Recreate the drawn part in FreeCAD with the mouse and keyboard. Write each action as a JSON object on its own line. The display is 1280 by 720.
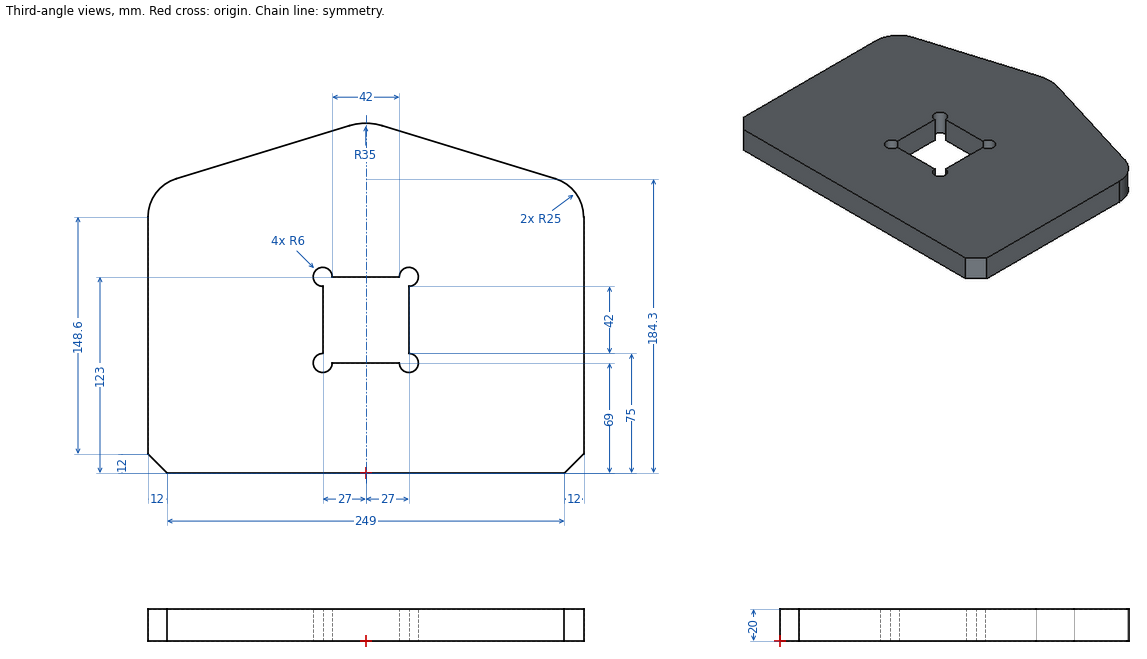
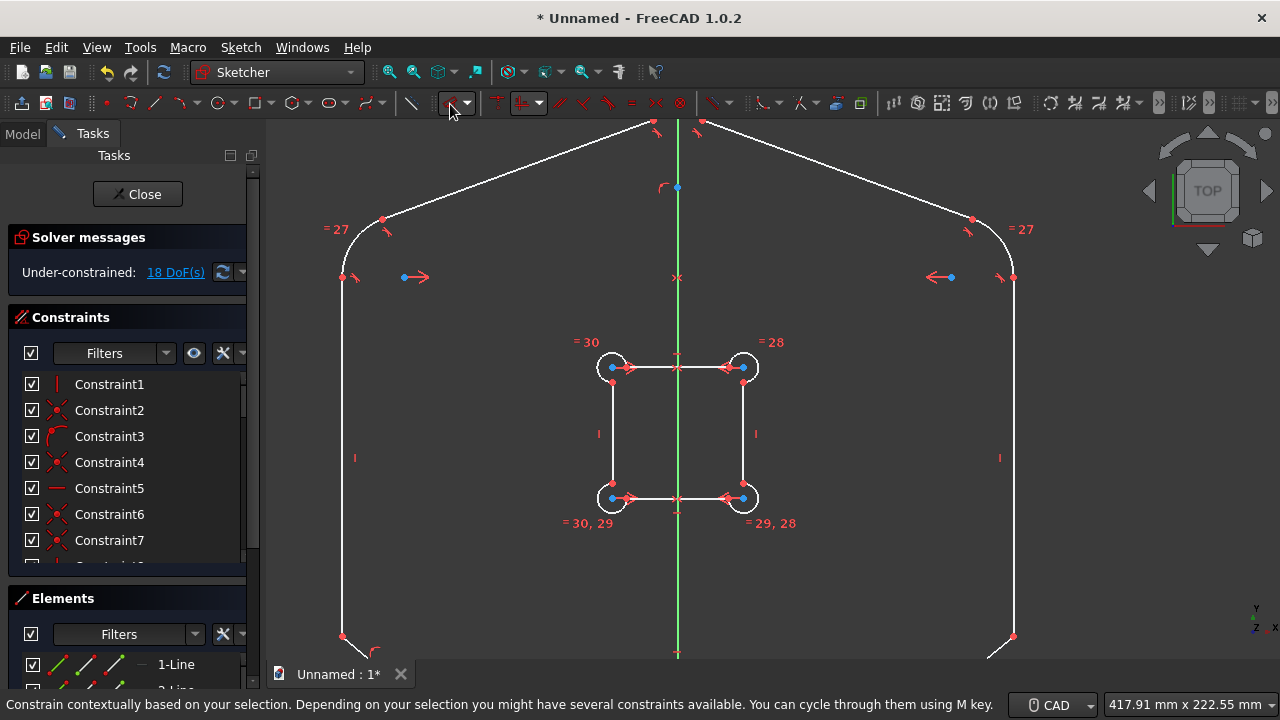
{"action": "scroll", "coordinate": [759, 369], "scroll_direction": "down", "scroll_amount": 2}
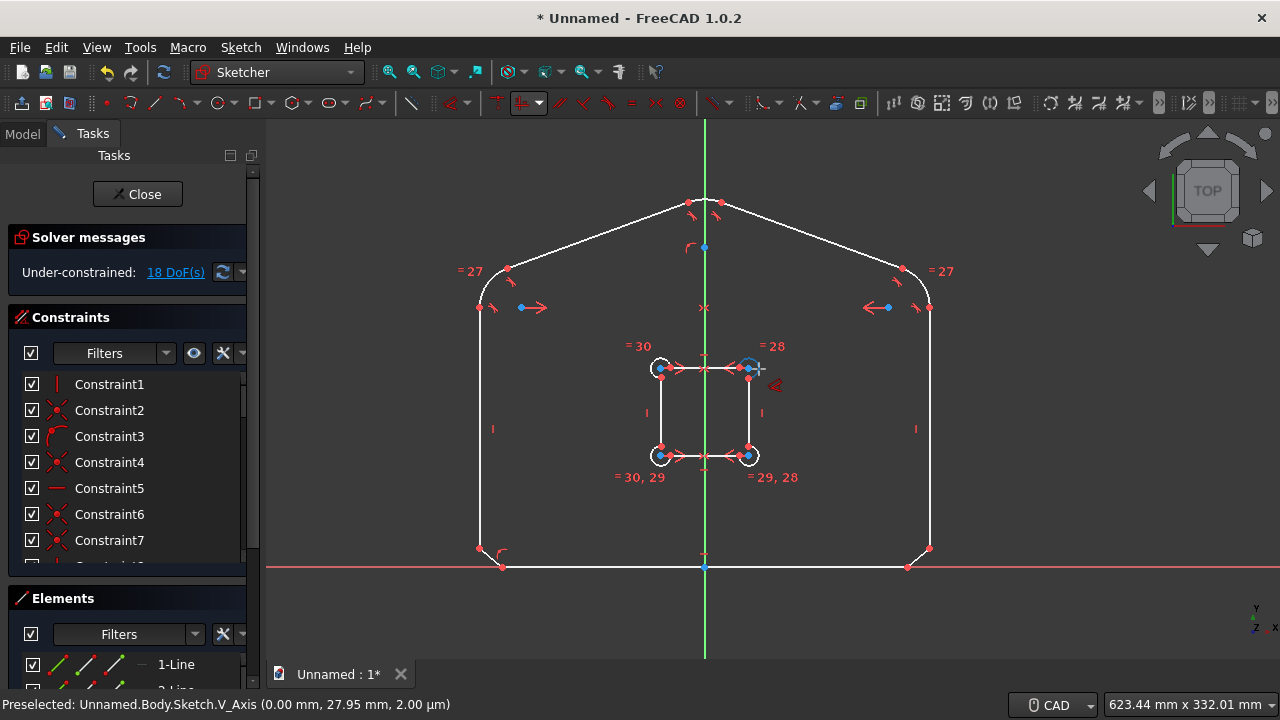
{"action": "scroll", "coordinate": [712, 200], "scroll_direction": "up", "scroll_amount": 4}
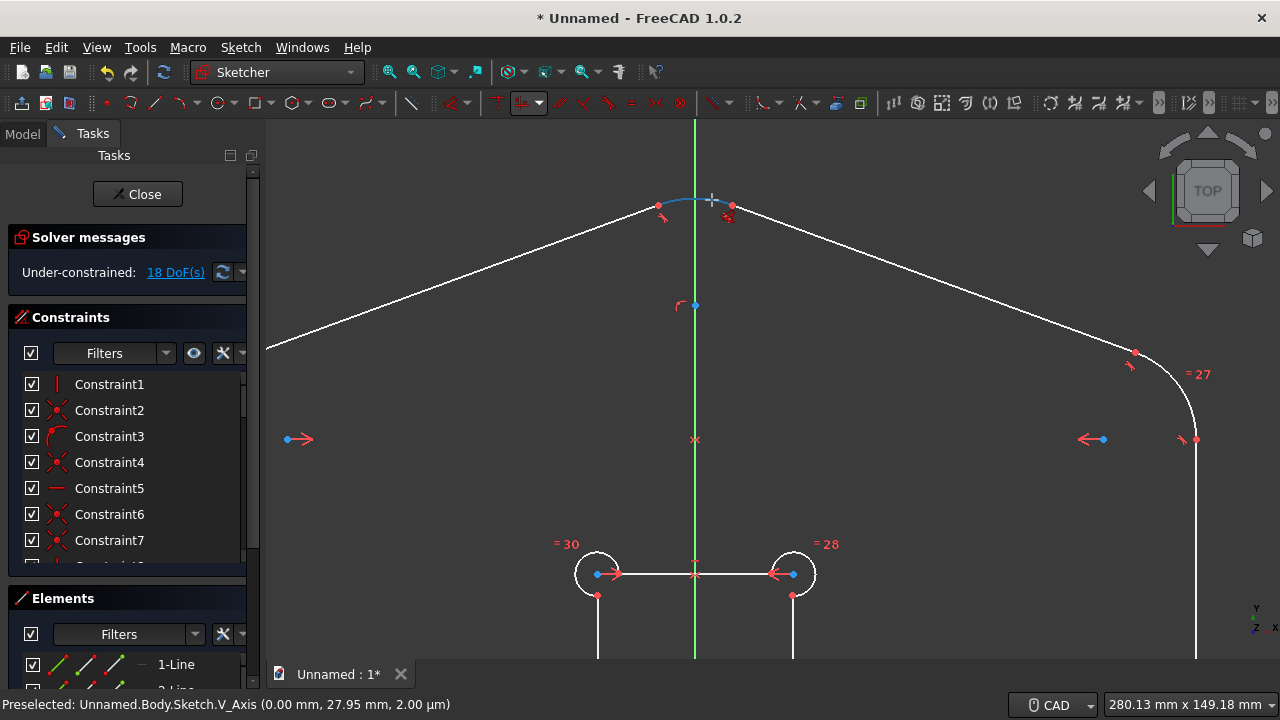
{"action": "left_click", "coordinate": [710, 200]}
{"action": "left_click", "coordinate": [714, 168]}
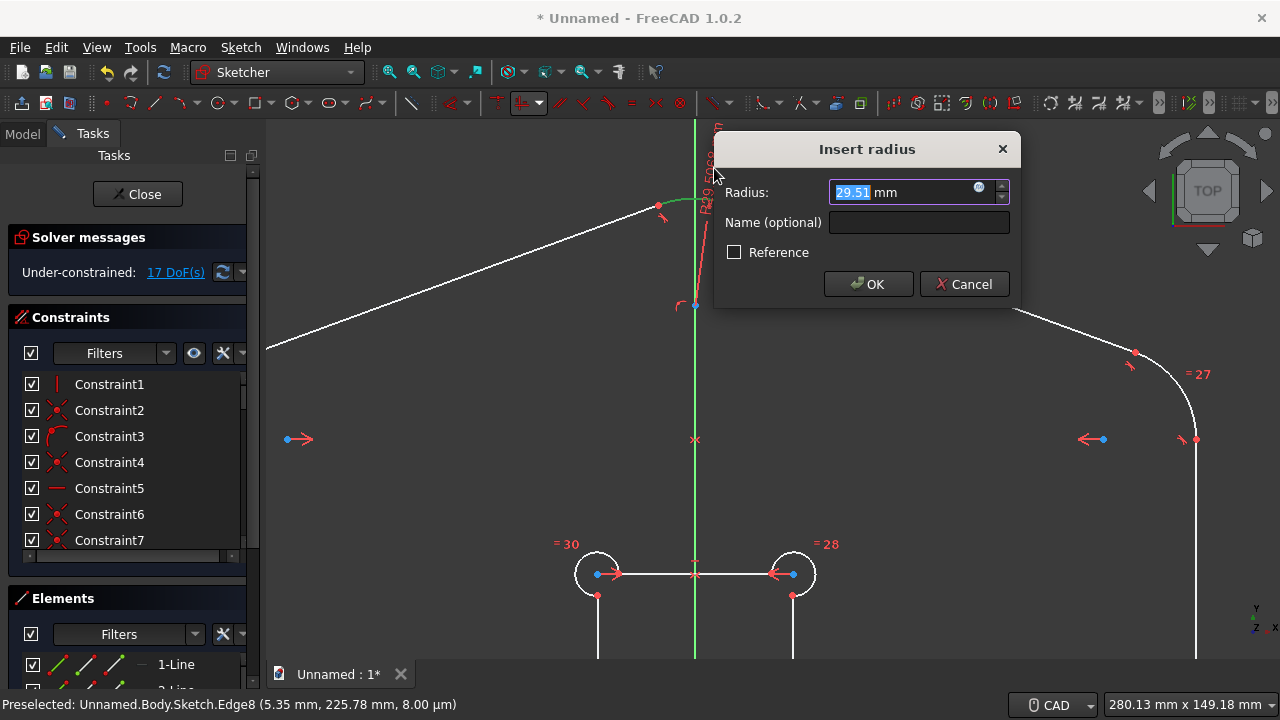
{"action": "type", "text": "35"}
{"action": "key", "text": "Return"}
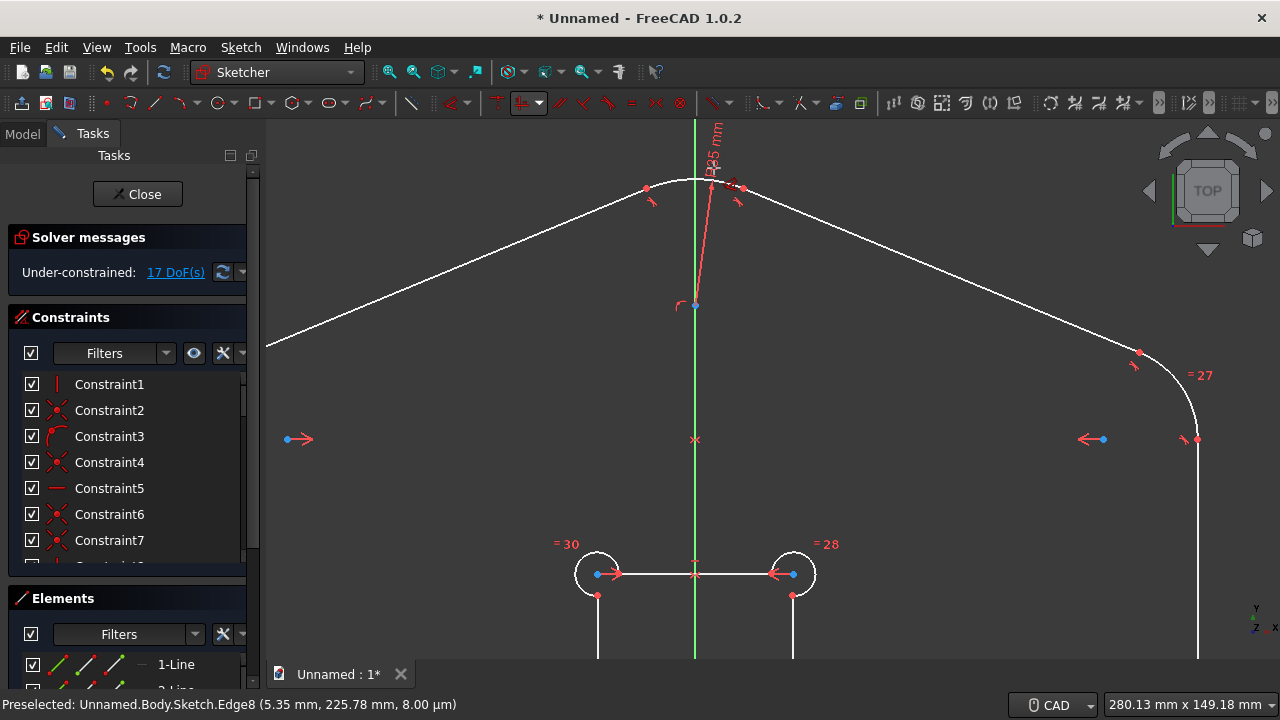
{"action": "scroll", "coordinate": [712, 200], "scroll_direction": "down", "scroll_amount": 4}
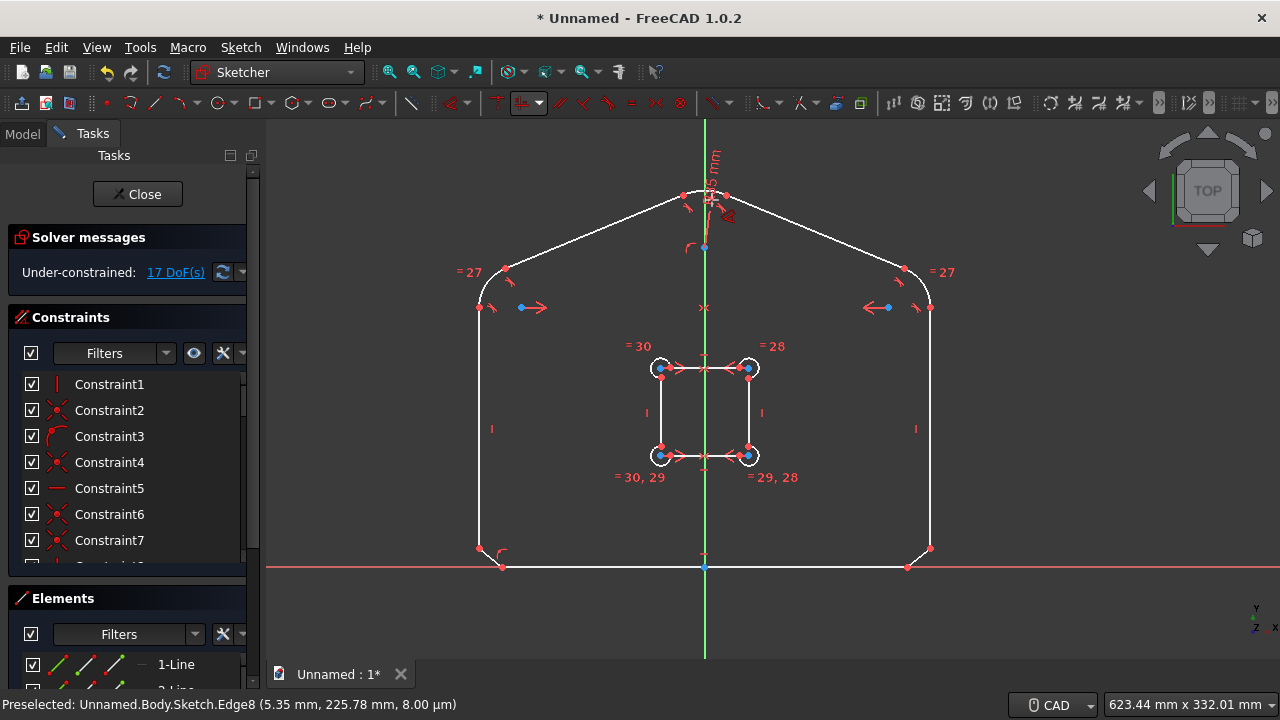
{"action": "left_click", "coordinate": [493, 277]}
{"action": "left_click", "coordinate": [471, 253]}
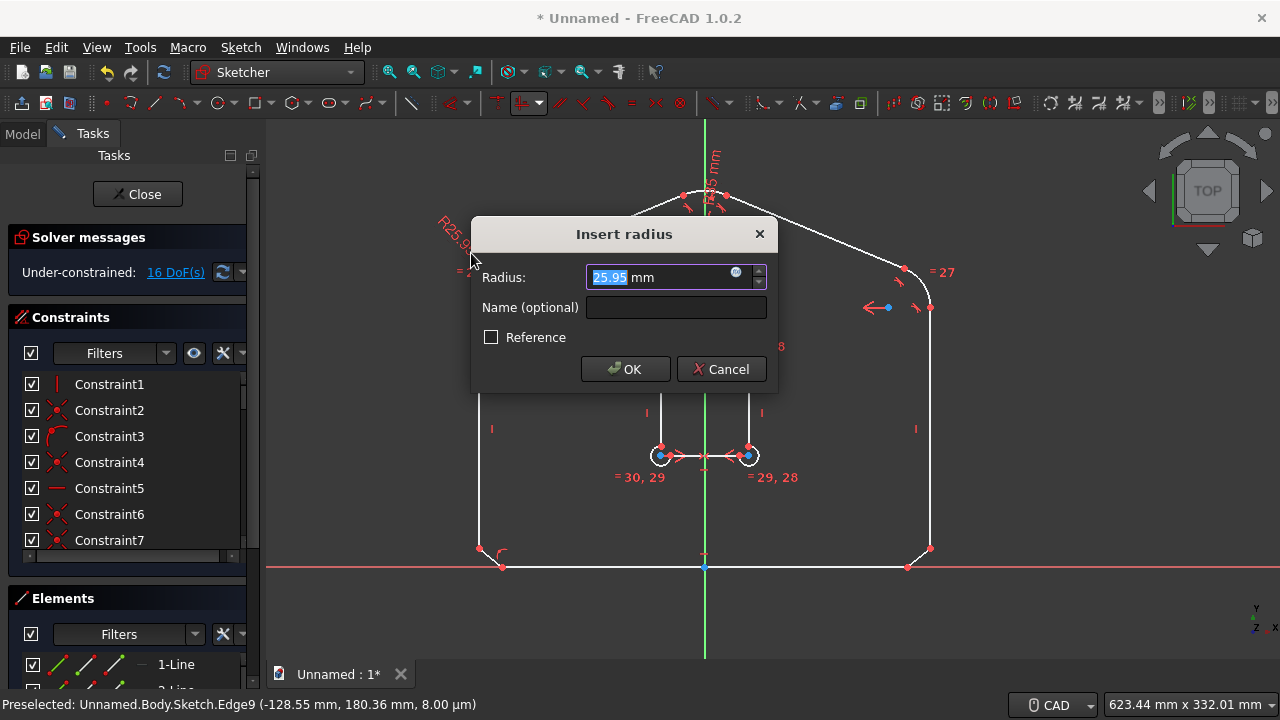
{"action": "type", "text": "25"}
{"action": "key", "text": "Return"}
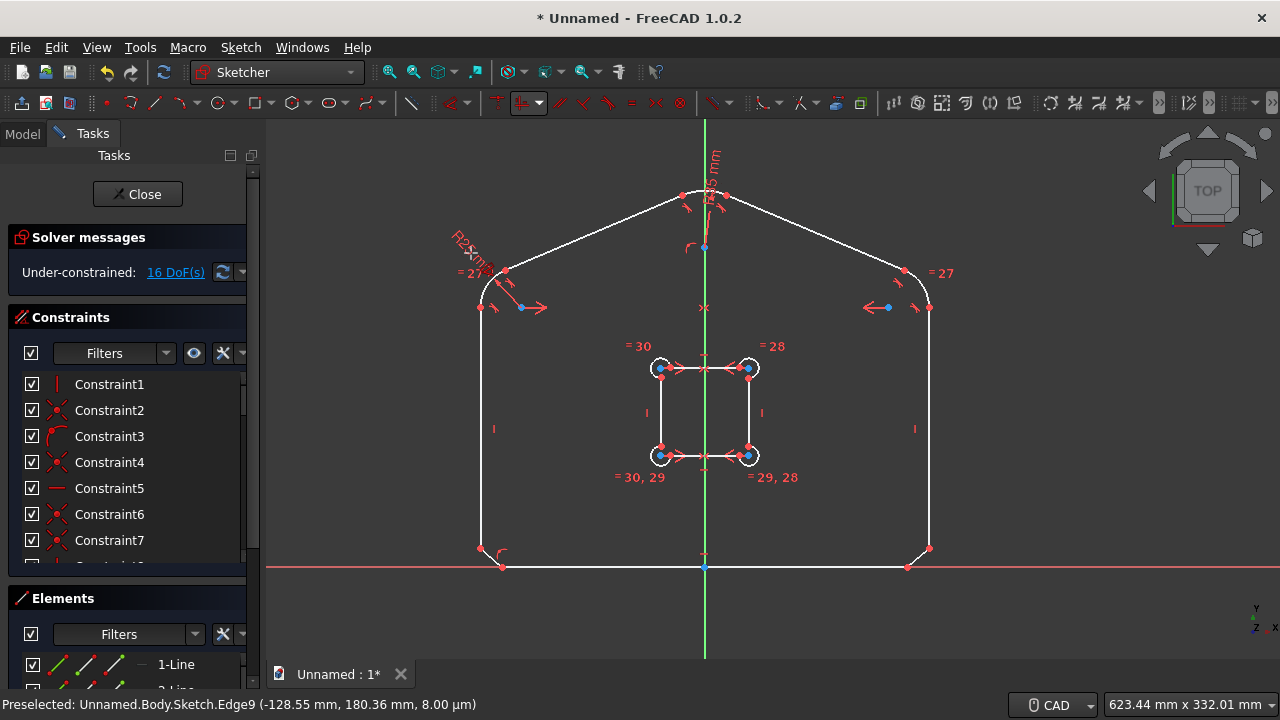
{"action": "scroll", "coordinate": [759, 370], "scroll_direction": "up", "scroll_amount": 8}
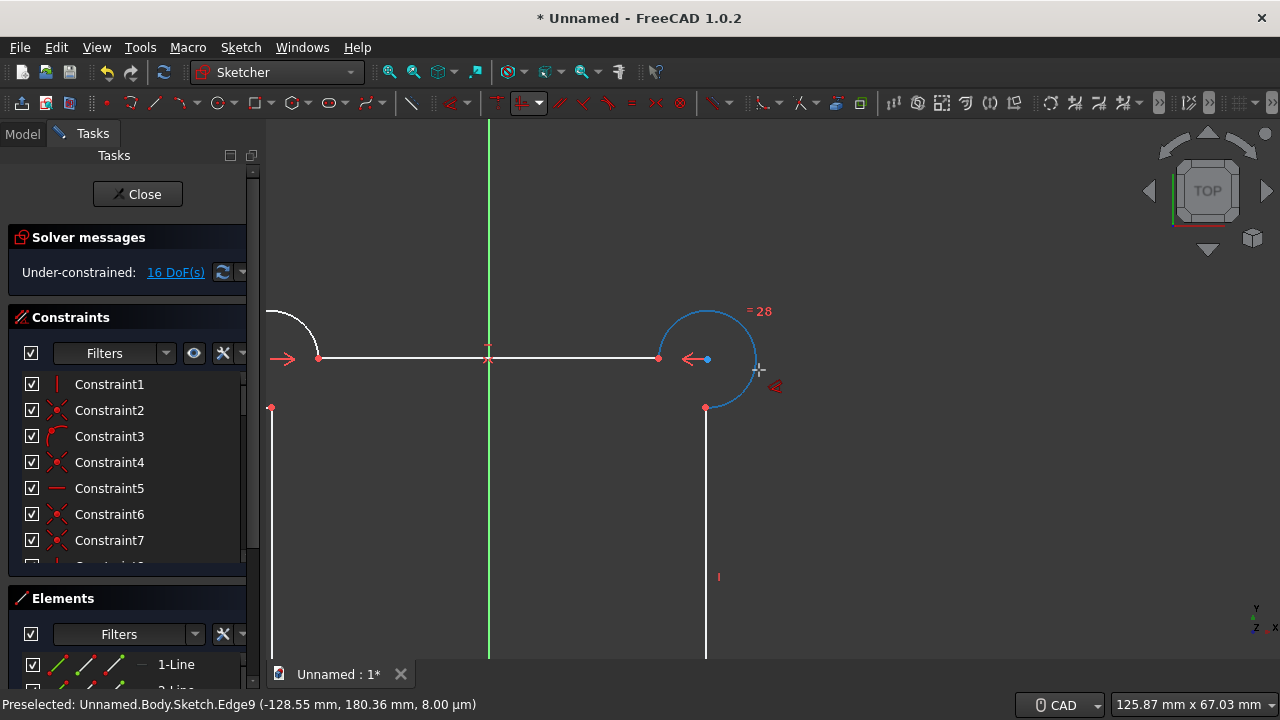
{"action": "left_click", "coordinate": [755, 368]}
{"action": "left_click", "coordinate": [786, 374]}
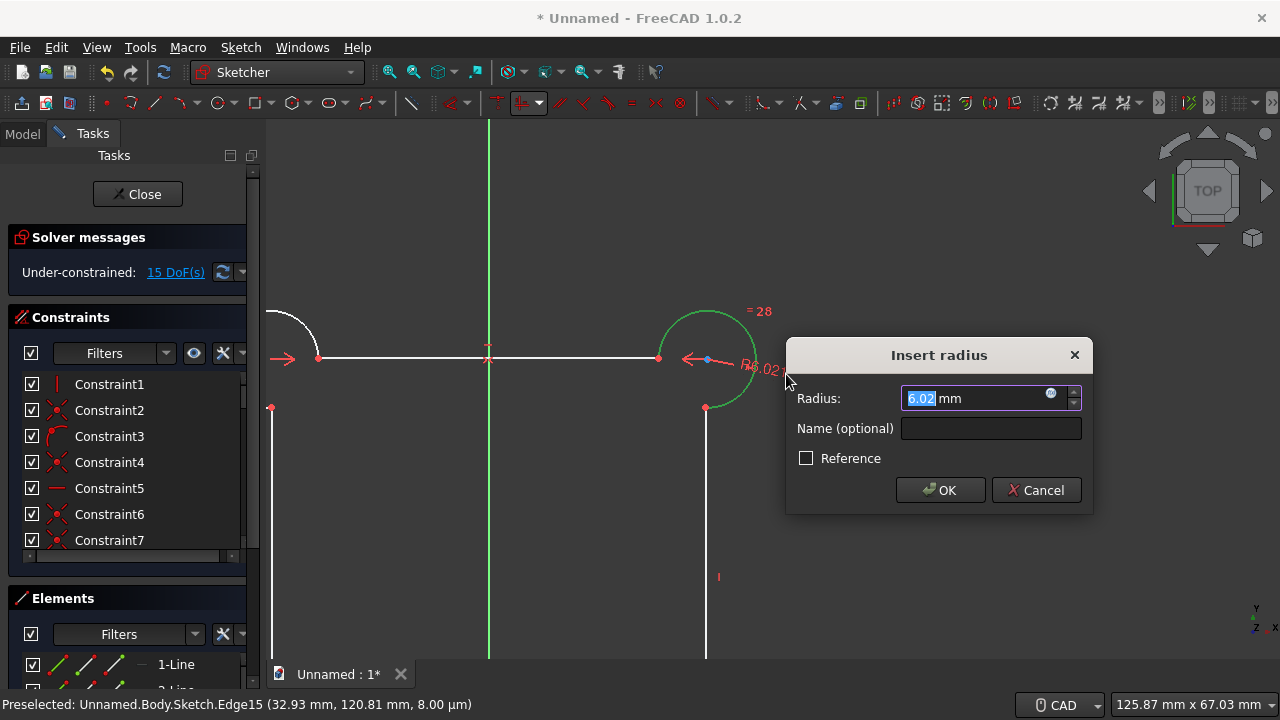
{"action": "type", "text": "6"}
{"action": "key", "text": "Return"}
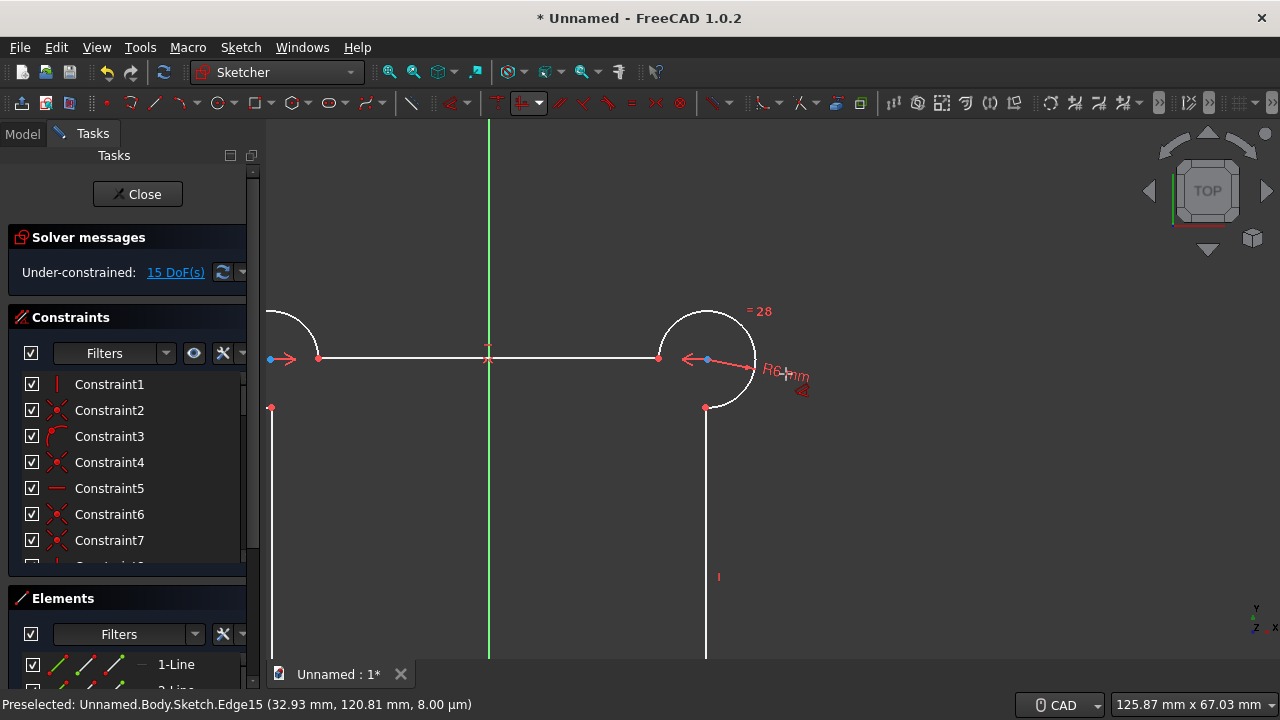
{"action": "scroll", "coordinate": [759, 370], "scroll_direction": "down", "scroll_amount": 8}